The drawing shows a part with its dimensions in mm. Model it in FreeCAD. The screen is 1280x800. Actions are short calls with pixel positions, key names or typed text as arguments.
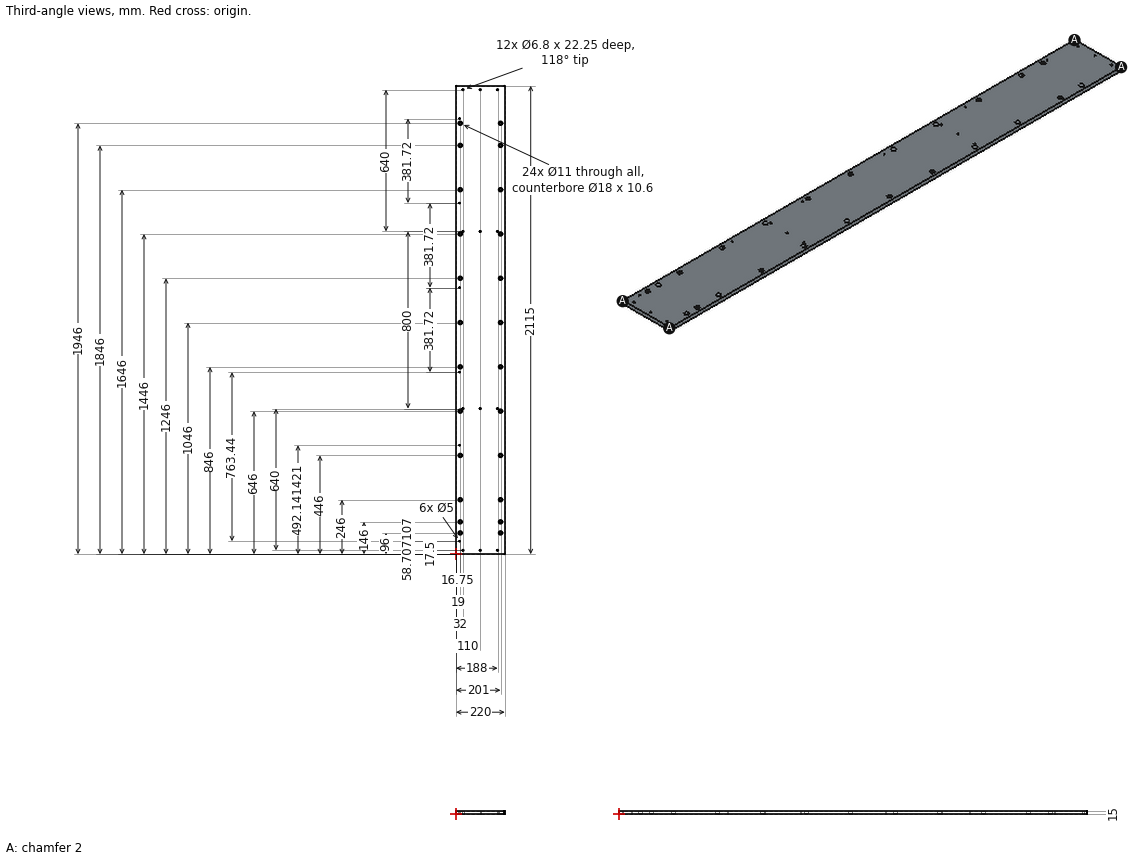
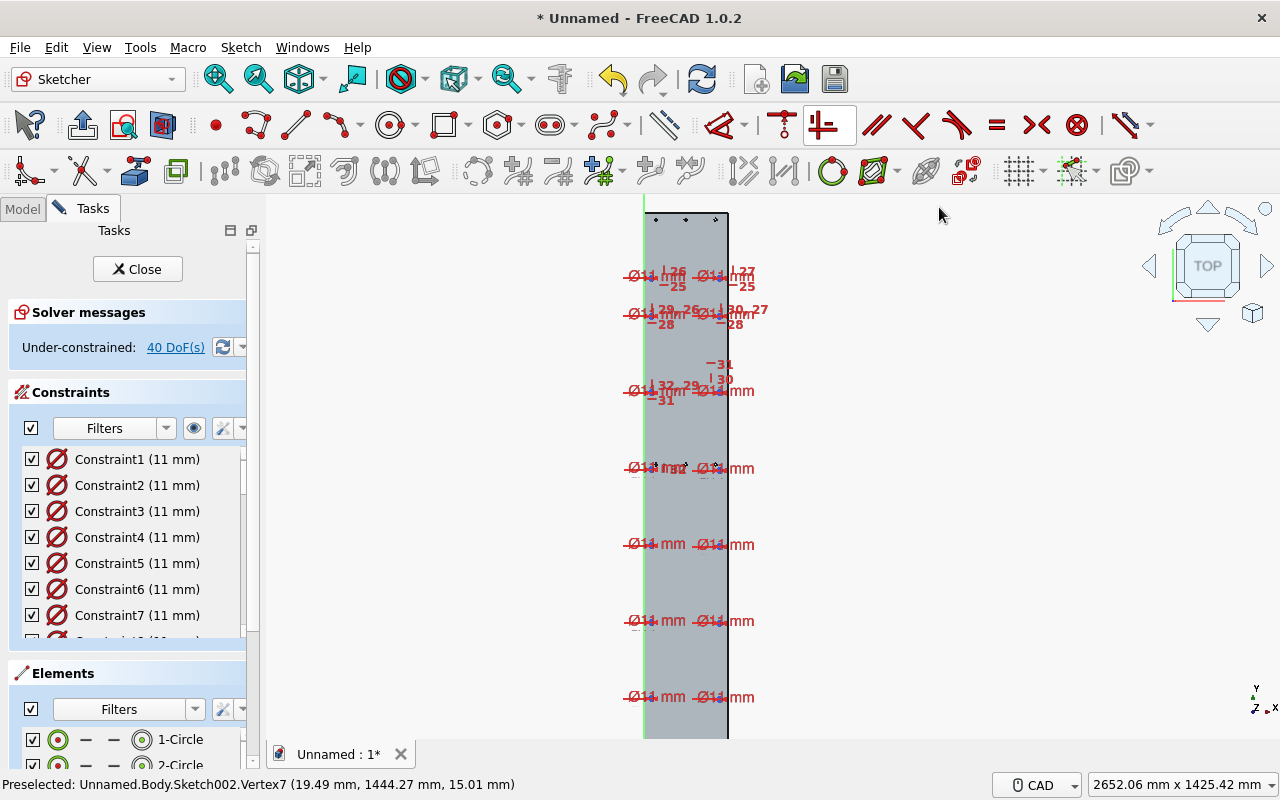
click(720, 393)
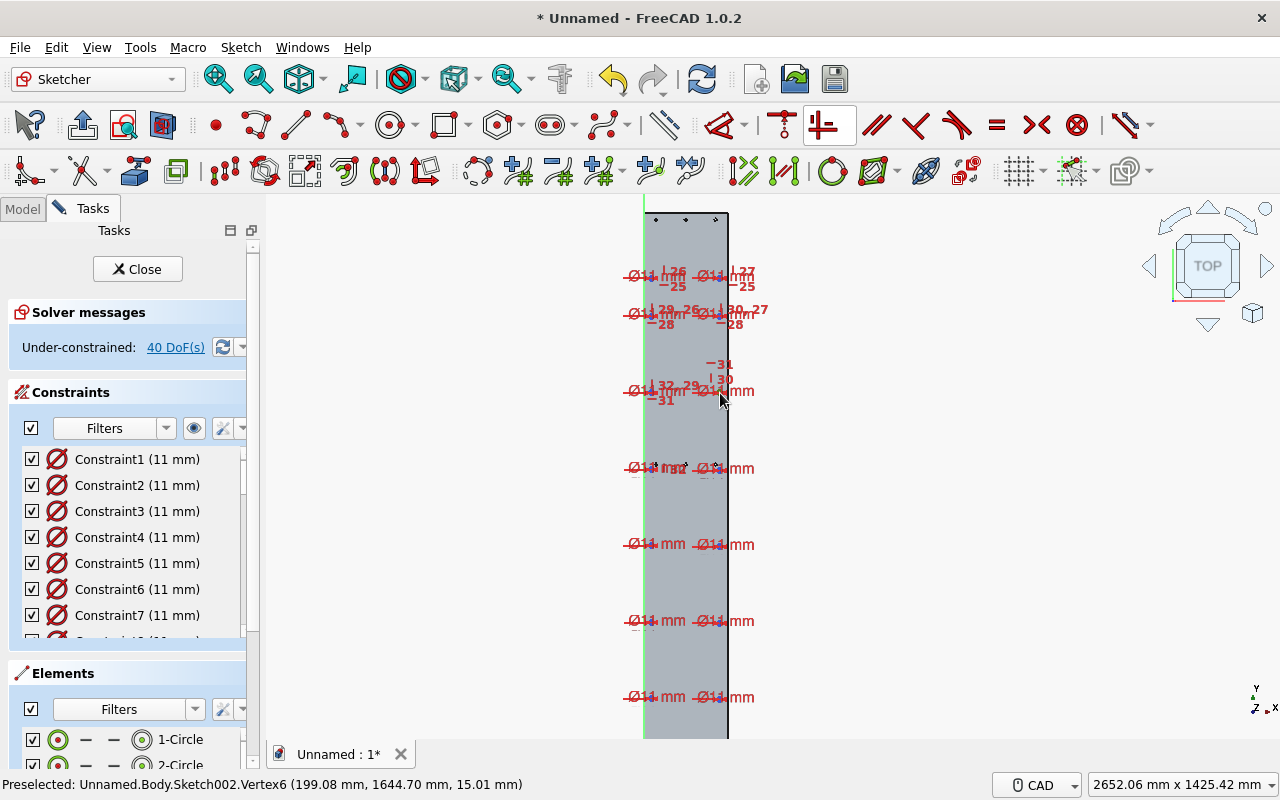
click(720, 471)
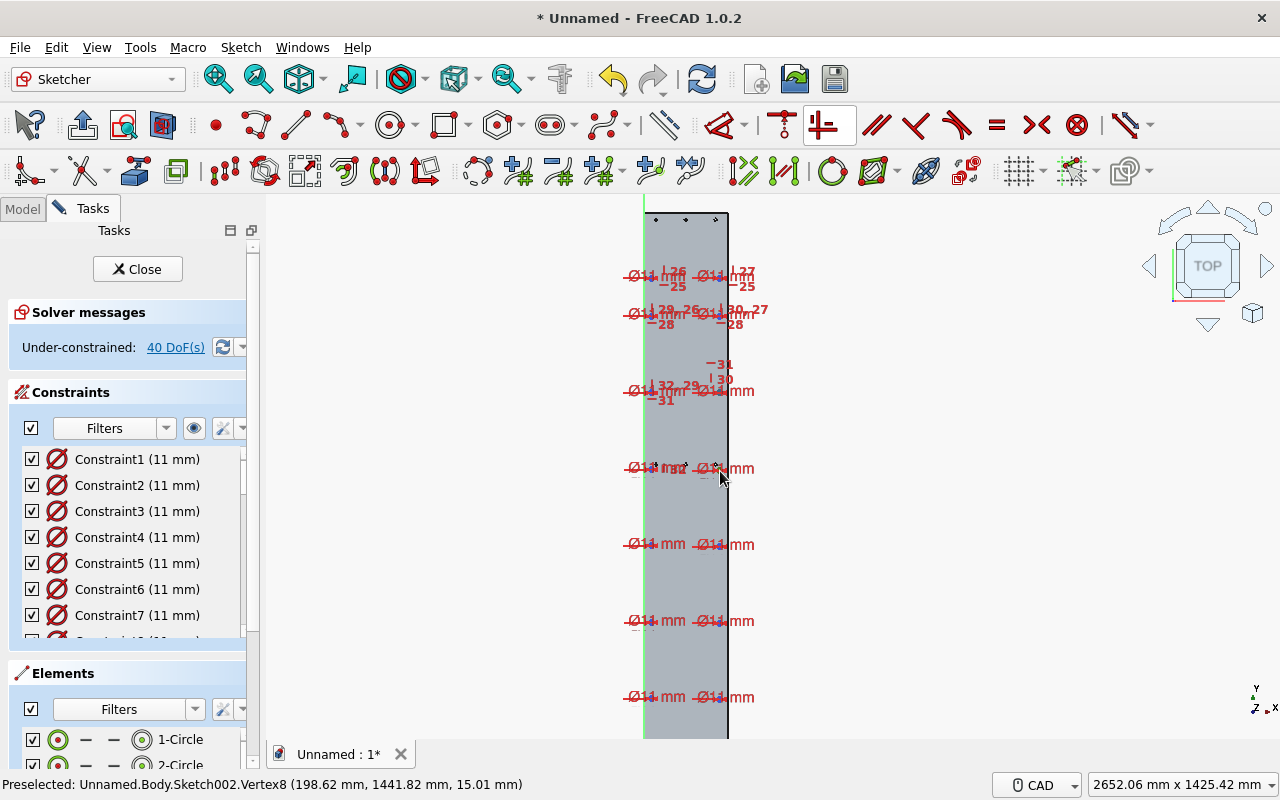
click(850, 126)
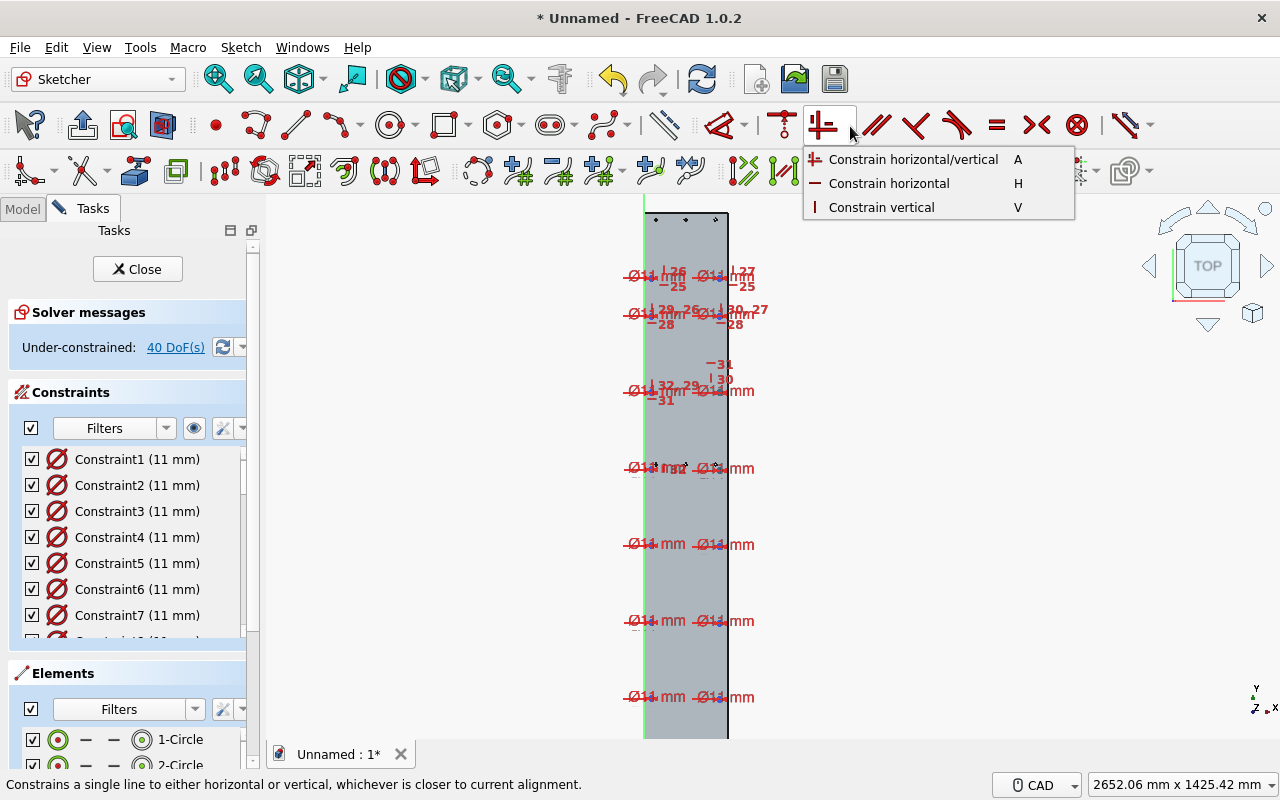
click(939, 207)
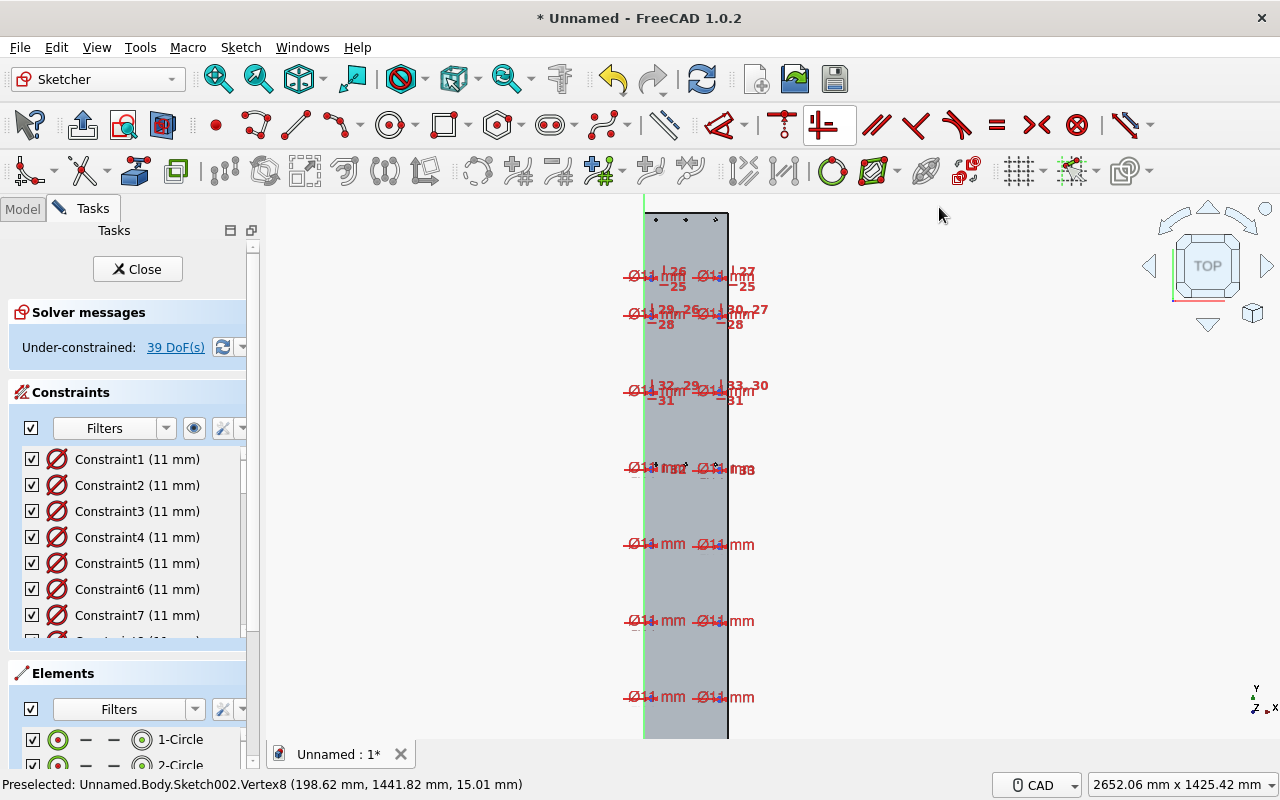
click(651, 470)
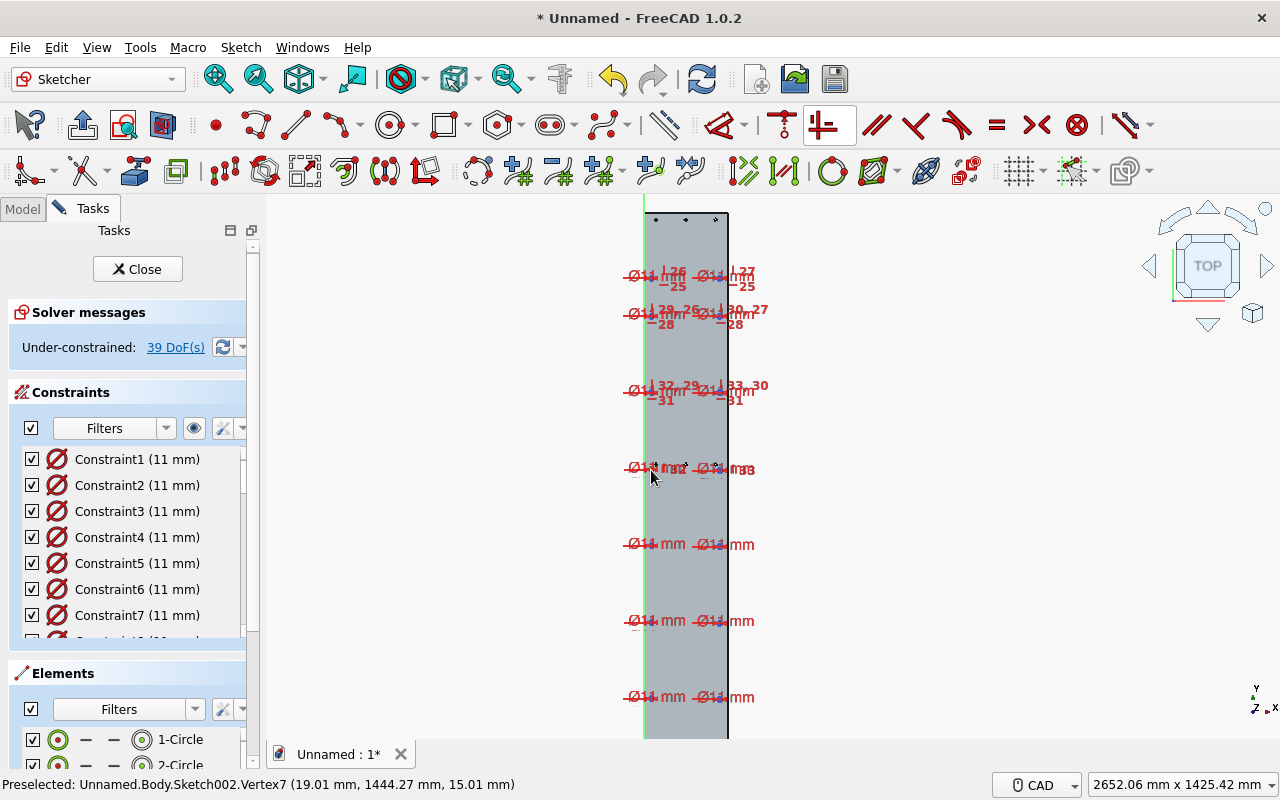
click(720, 471)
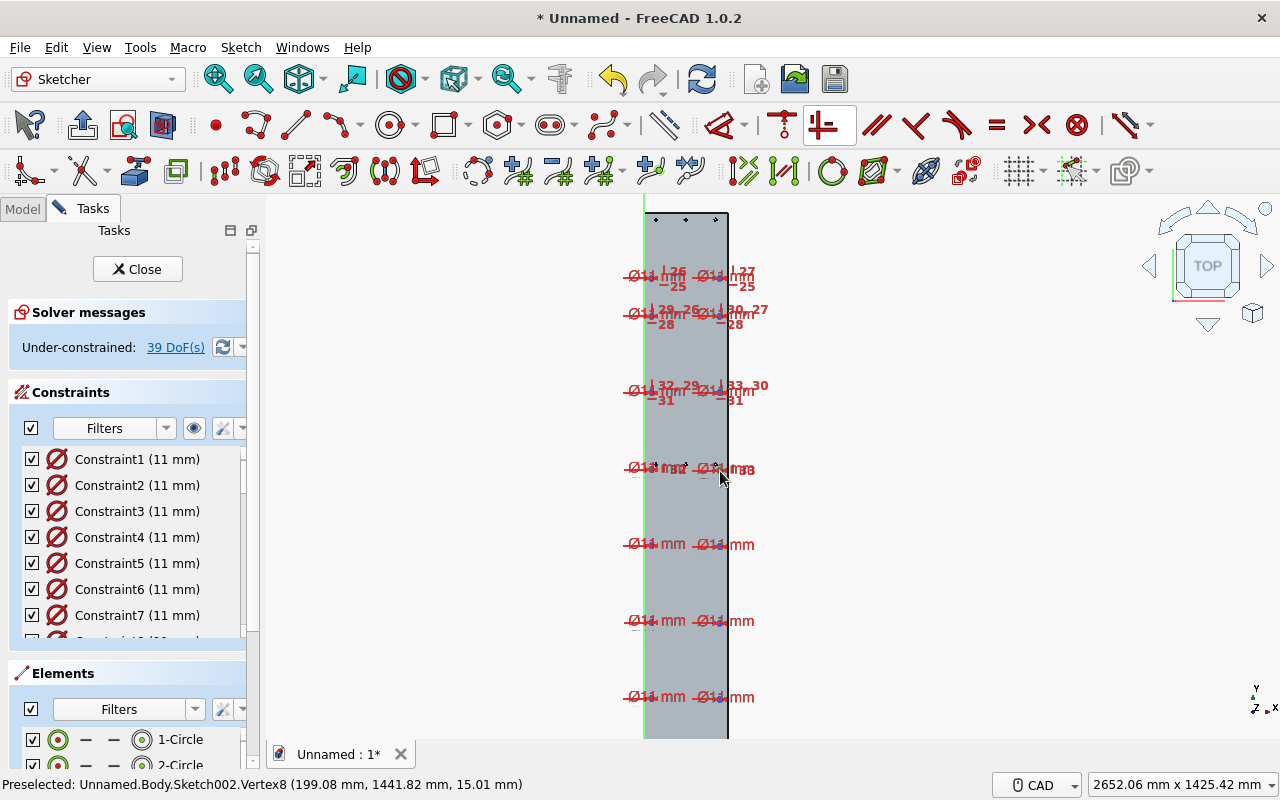
key(h)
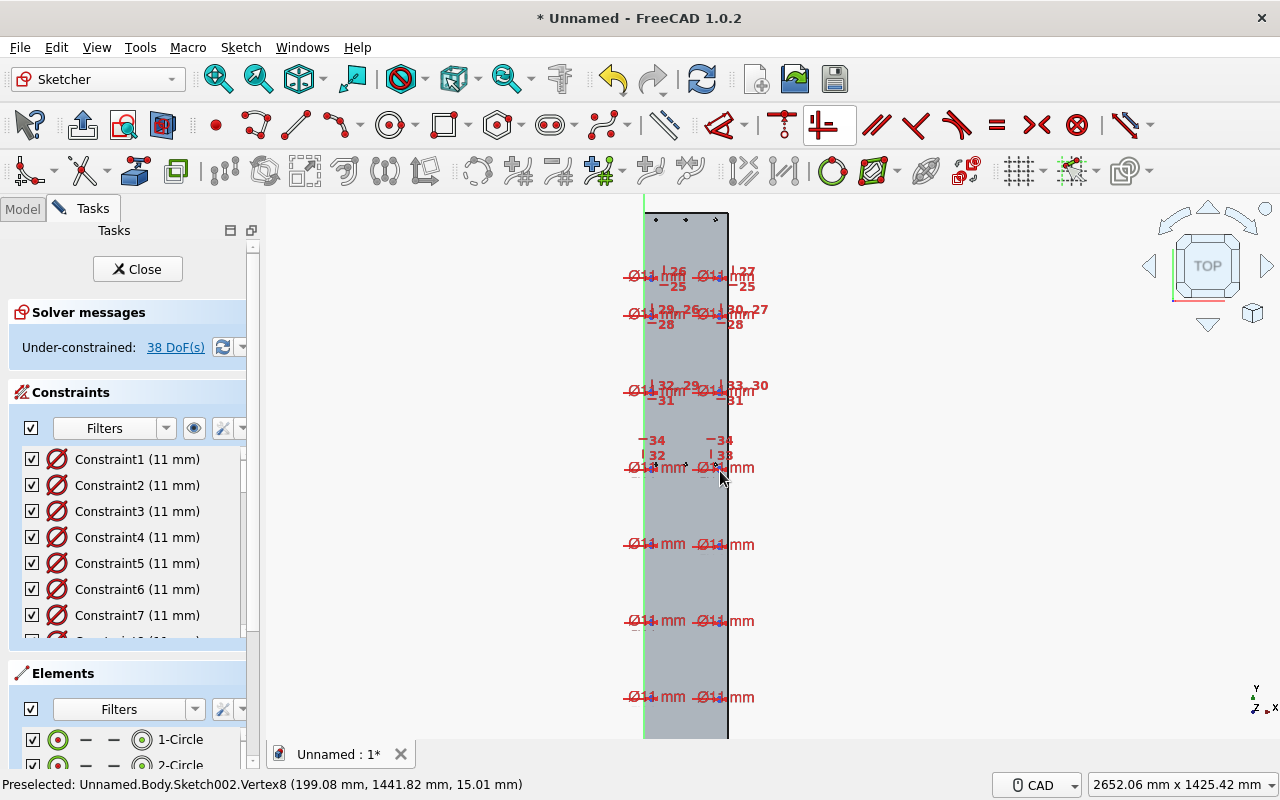
click(651, 470)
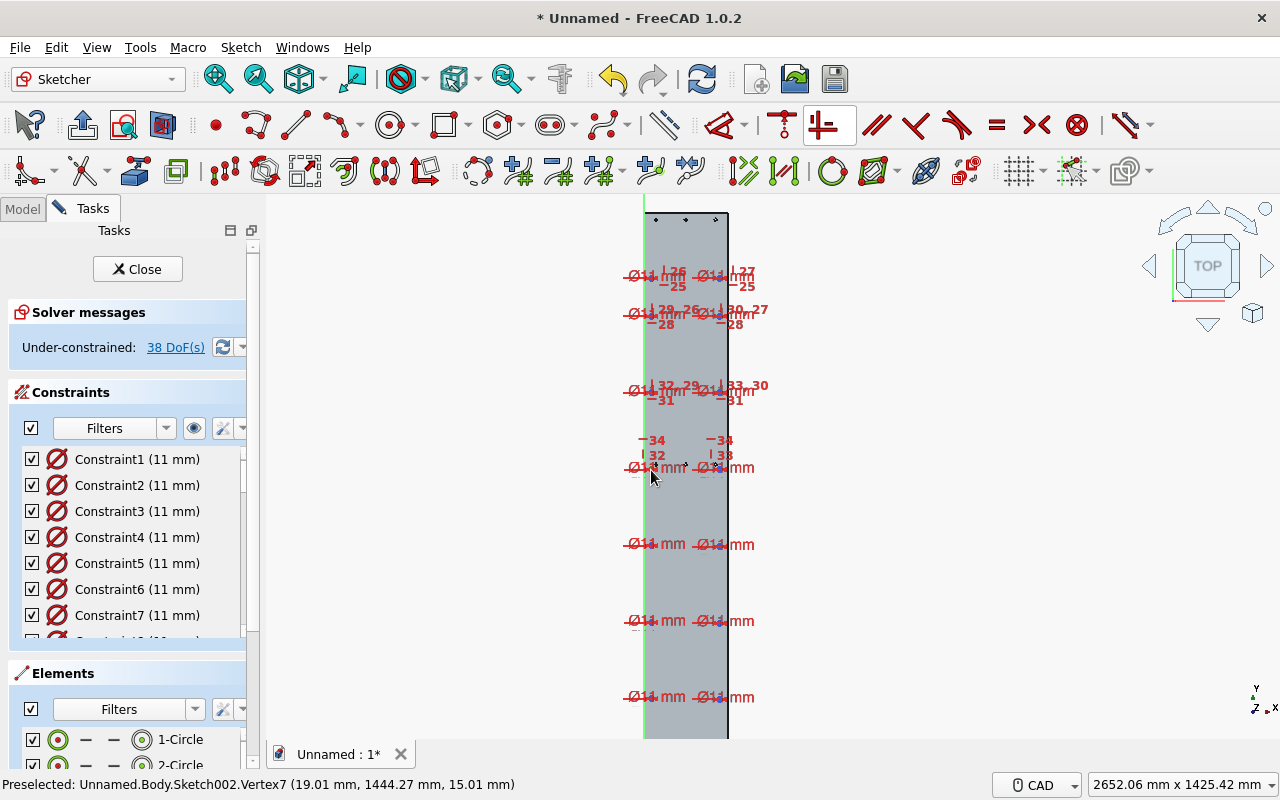
click(651, 546)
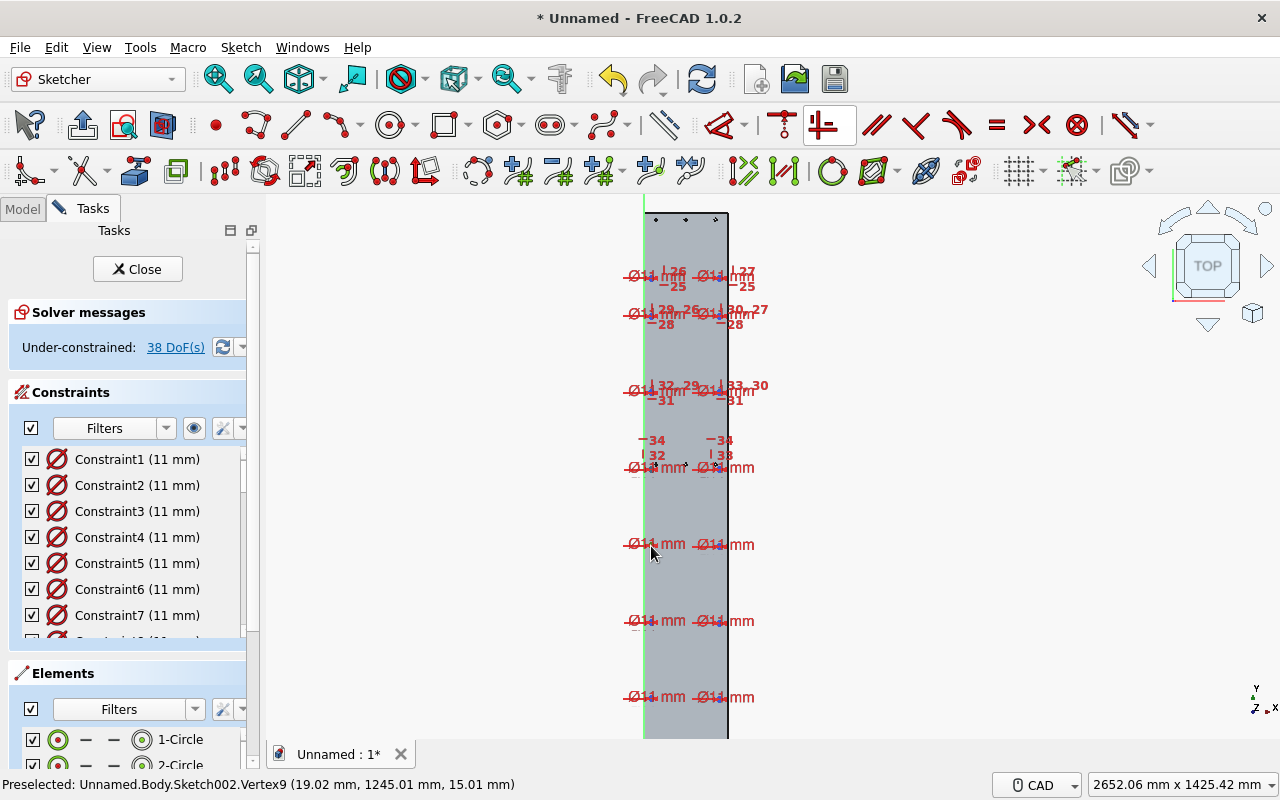
key(v)